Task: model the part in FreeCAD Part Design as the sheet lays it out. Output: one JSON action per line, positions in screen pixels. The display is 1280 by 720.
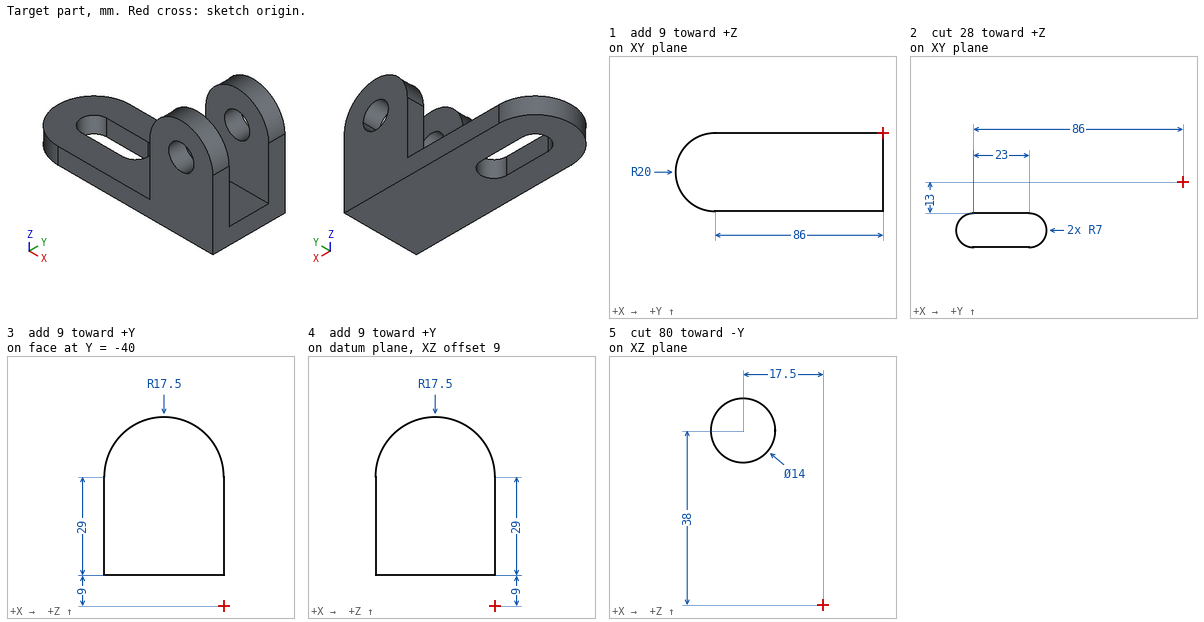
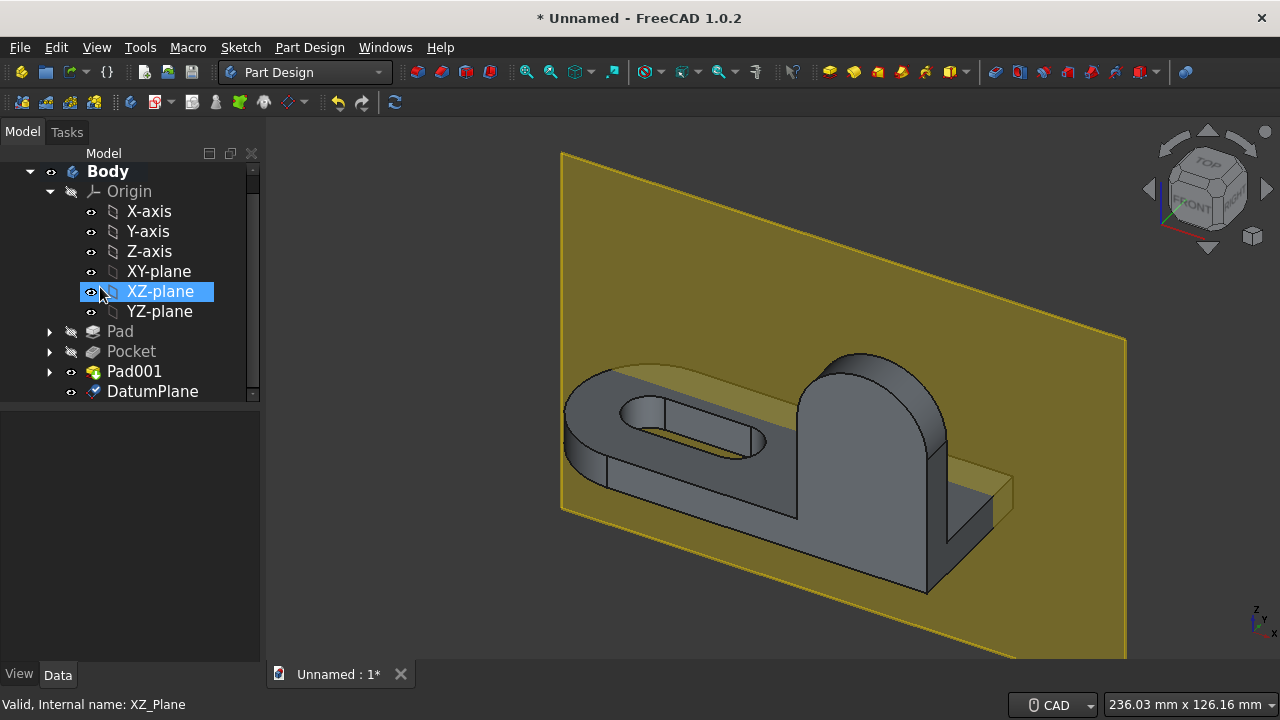
{"action": "left_click", "coordinate": [116, 392]}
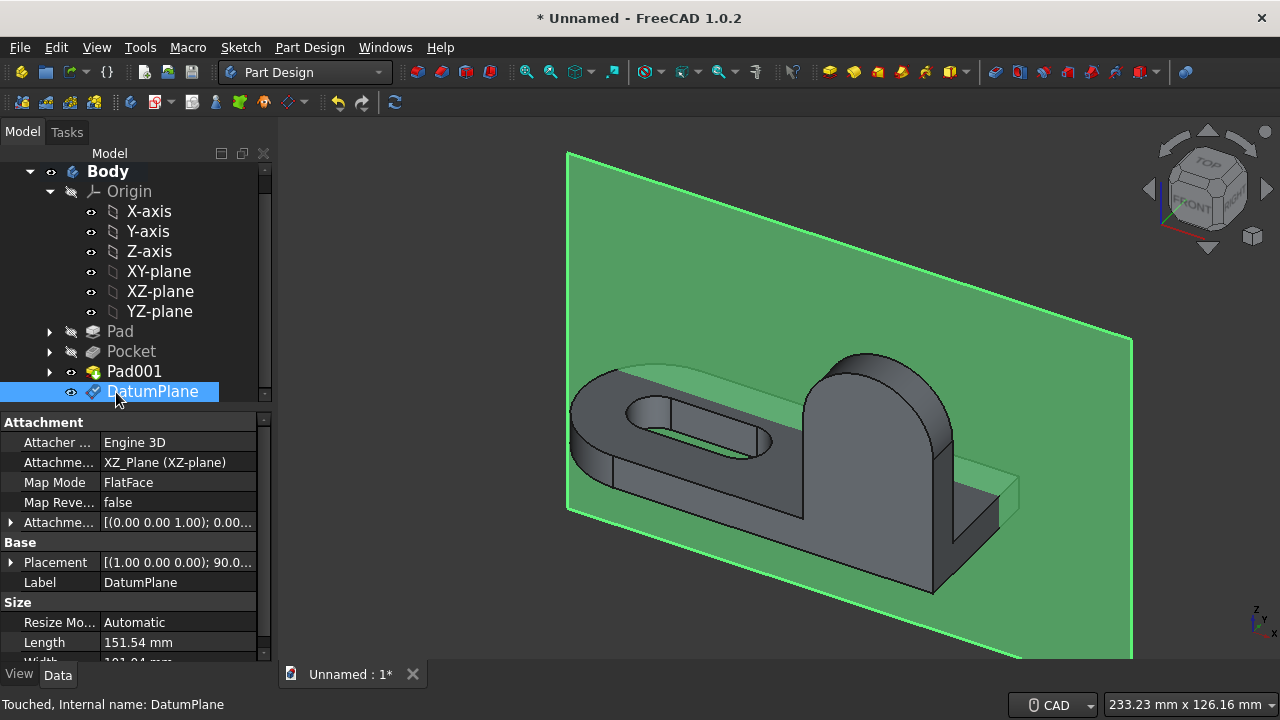
{"action": "left_click", "coordinate": [156, 102]}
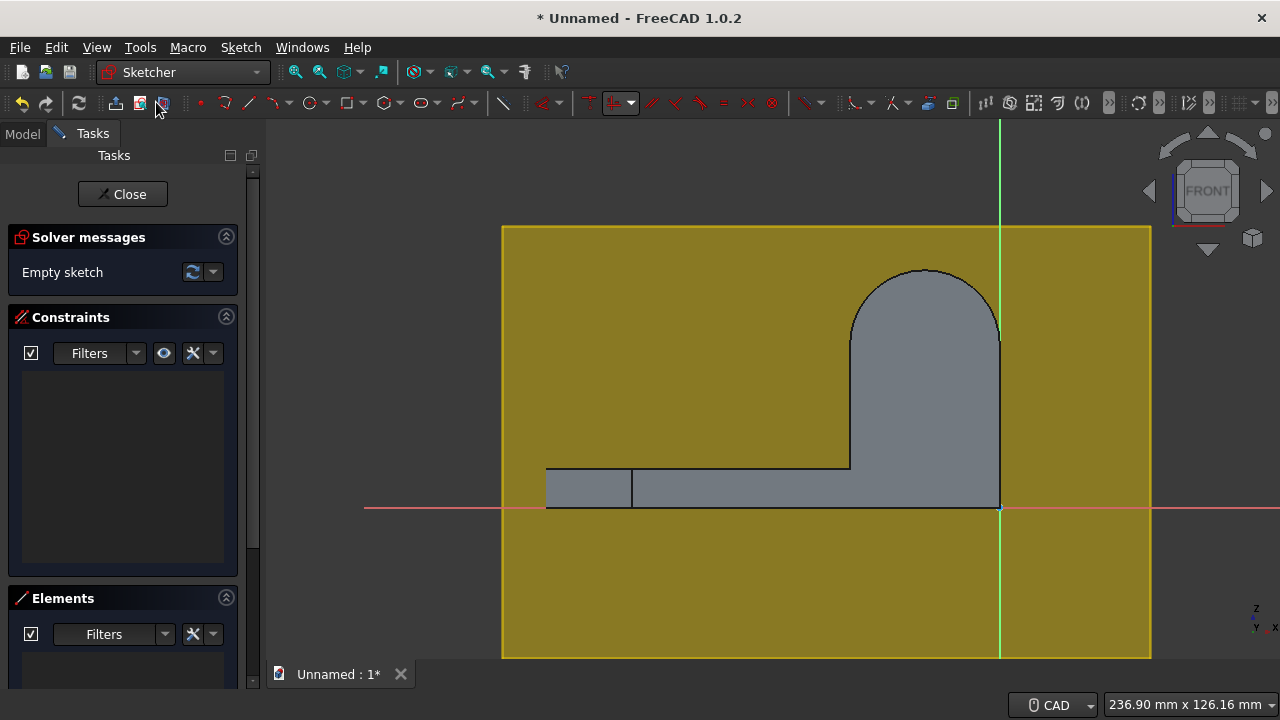
{"action": "left_click", "coordinate": [164, 104]}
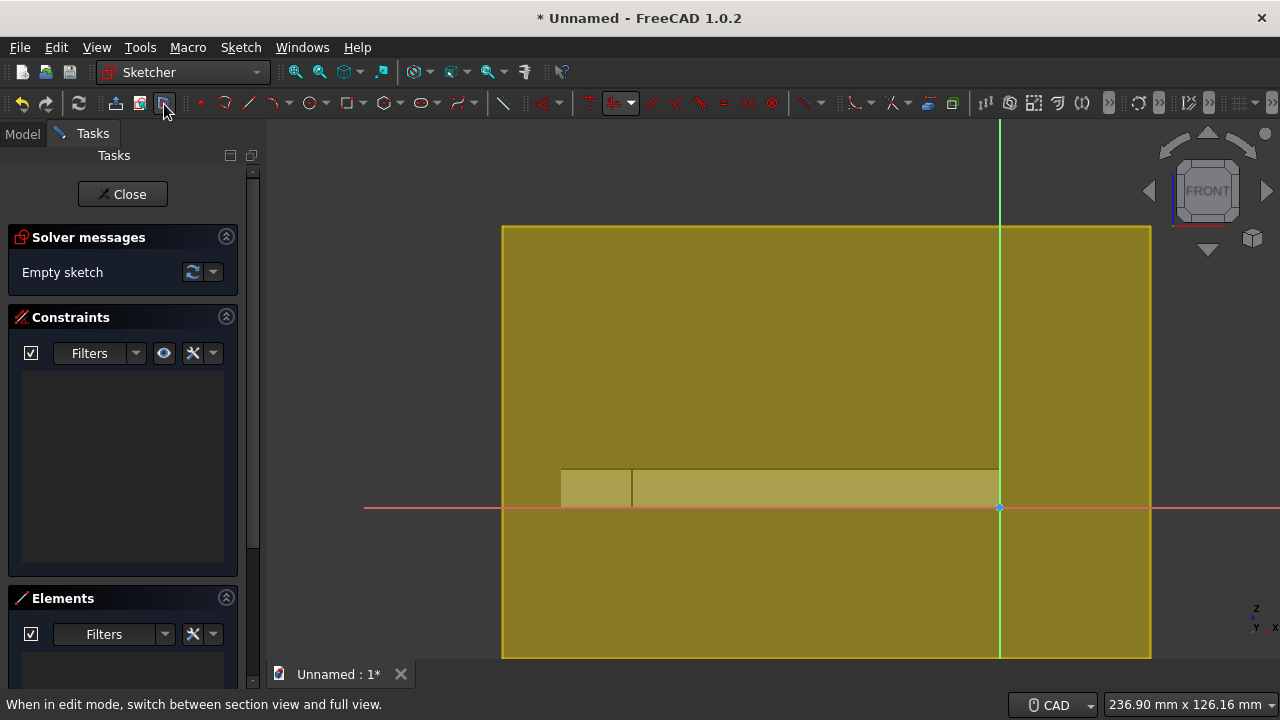
{"action": "scroll", "coordinate": [1115, 389], "scroll_direction": "up", "scroll_amount": 2}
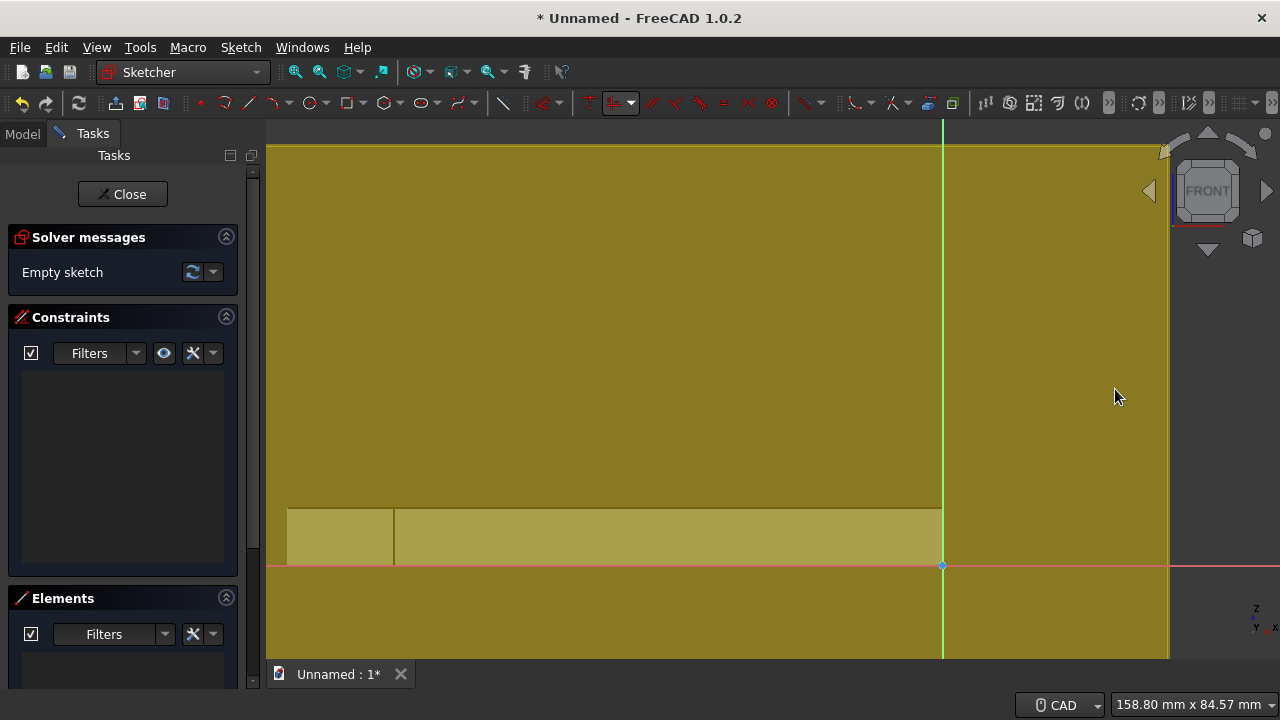
{"action": "left_click", "coordinate": [226, 104]}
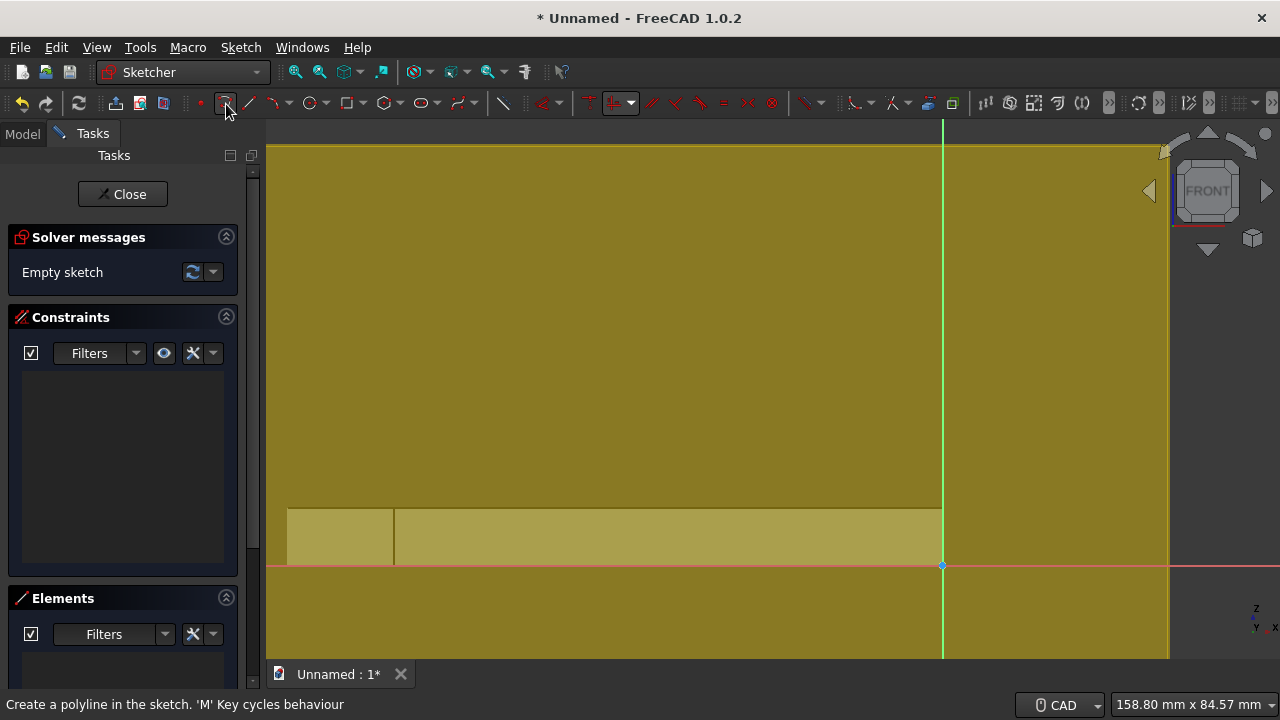
{"action": "left_click", "coordinate": [943, 323]}
{"action": "left_click", "coordinate": [934, 508]}
{"action": "left_click", "coordinate": [719, 508]}
{"action": "left_click", "coordinate": [719, 323]}
{"action": "right_click", "coordinate": [719, 323]}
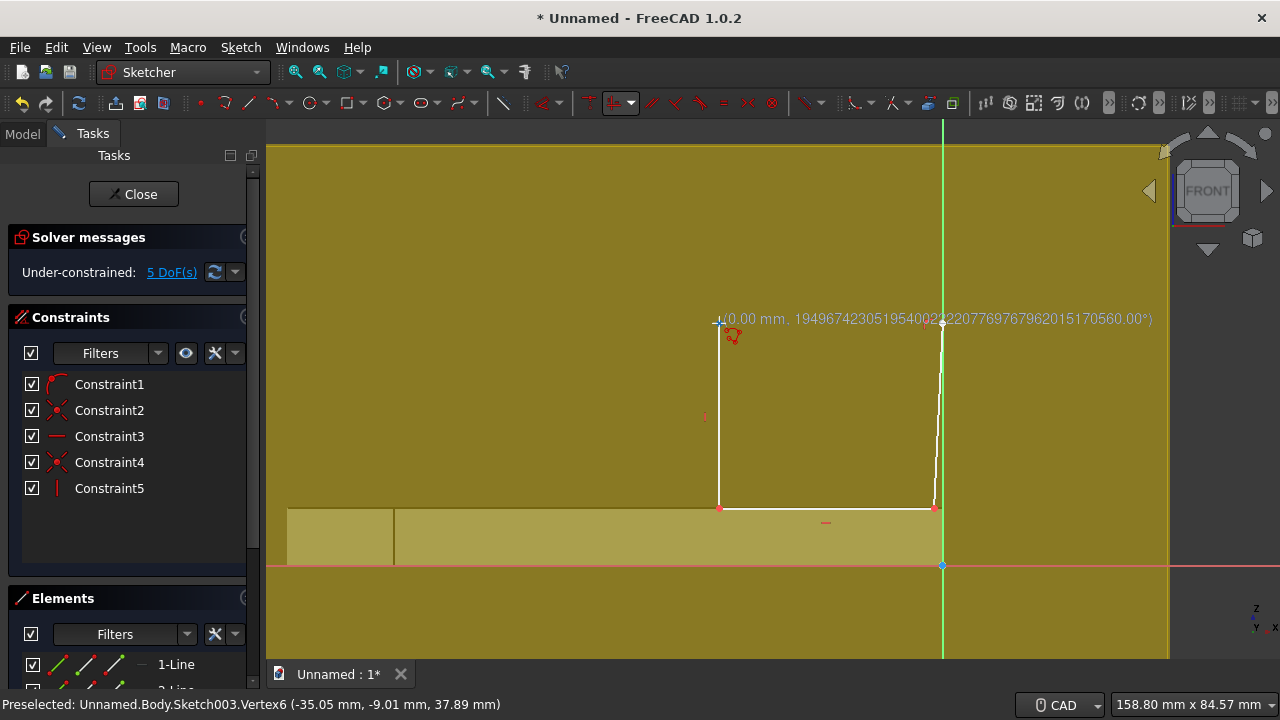
{"action": "left_click", "coordinate": [274, 104]}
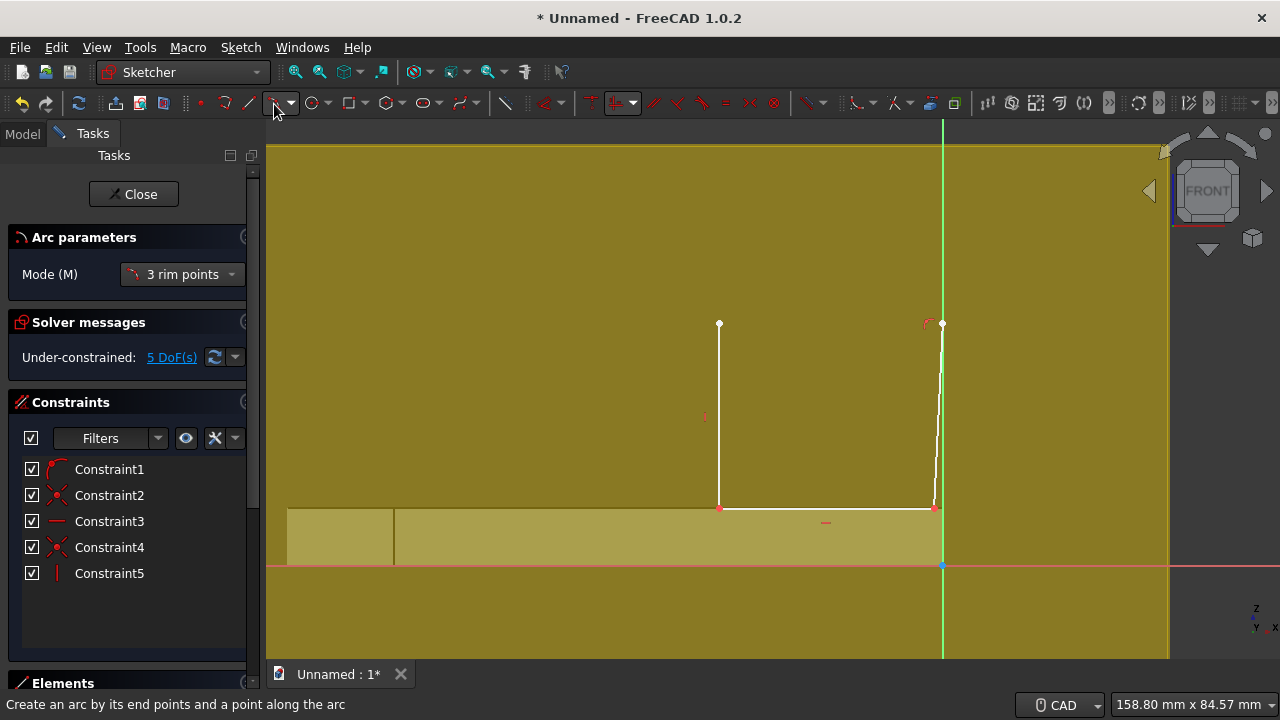
{"action": "left_click", "coordinate": [719, 324]}
{"action": "left_click", "coordinate": [943, 324]}
{"action": "left_click", "coordinate": [831, 212]}
{"action": "key", "text": "Escape"}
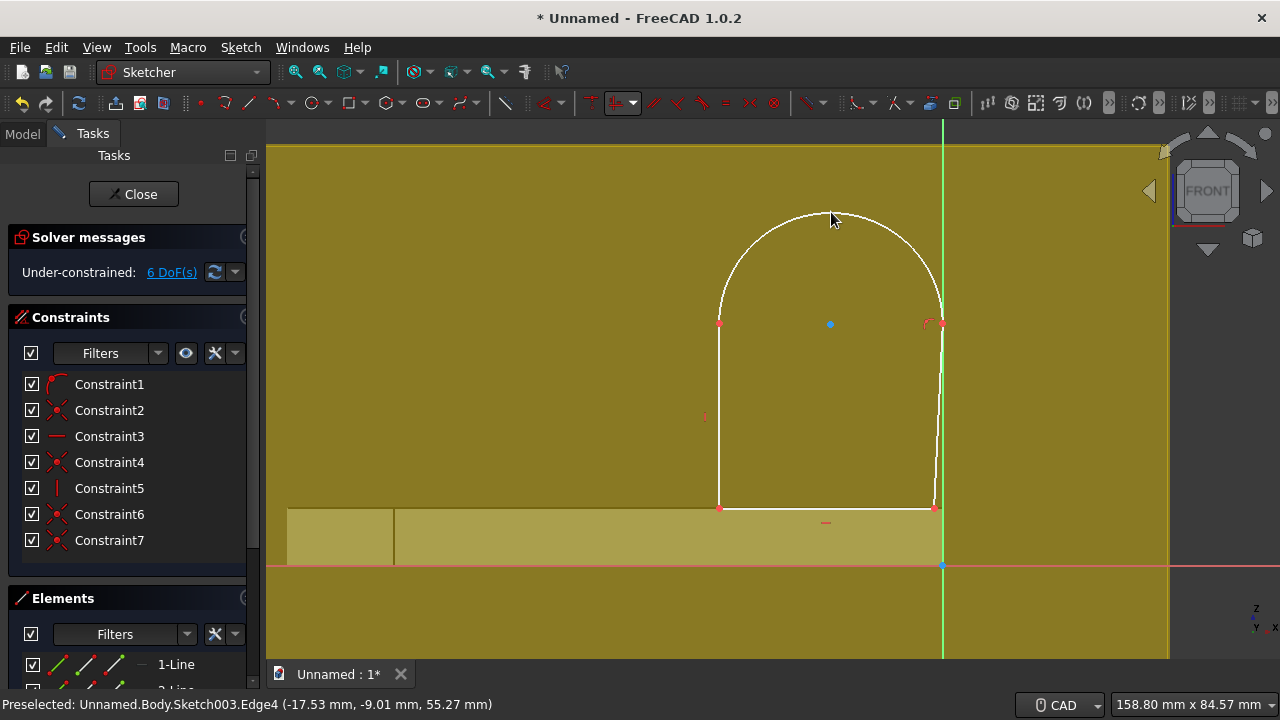
{"action": "left_click", "coordinate": [940, 379]}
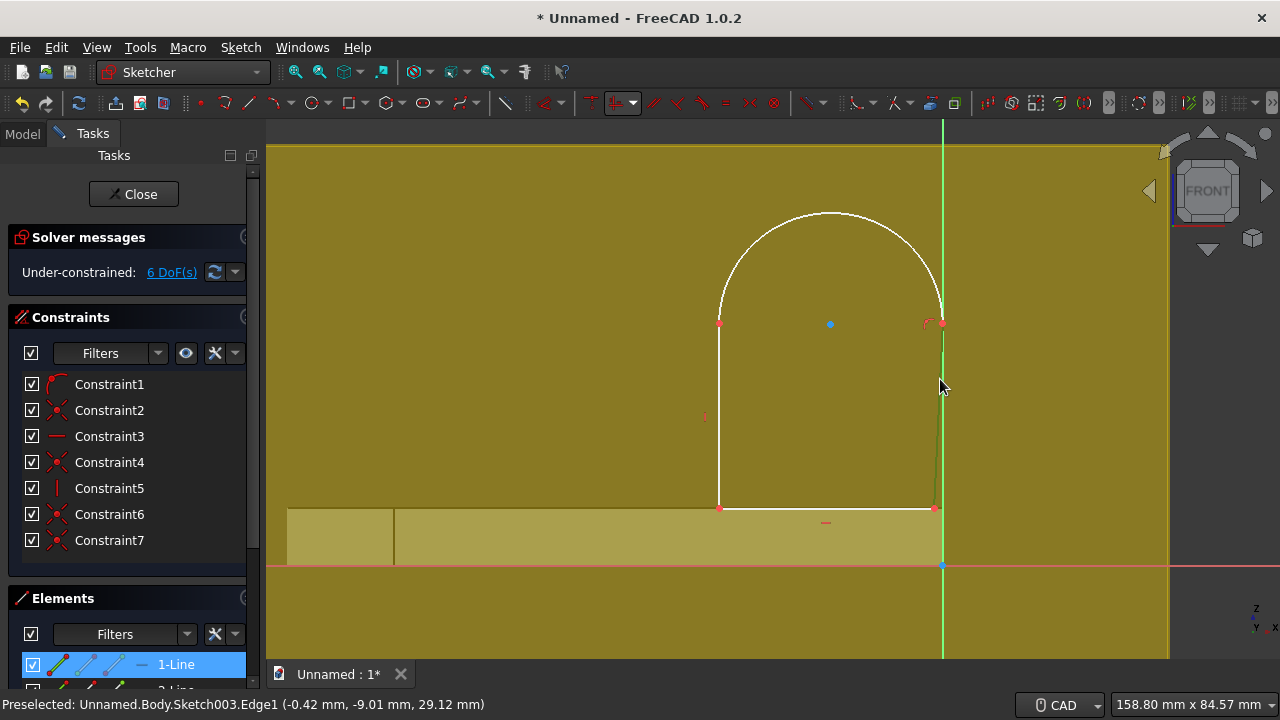
{"action": "left_click", "coordinate": [896, 234]}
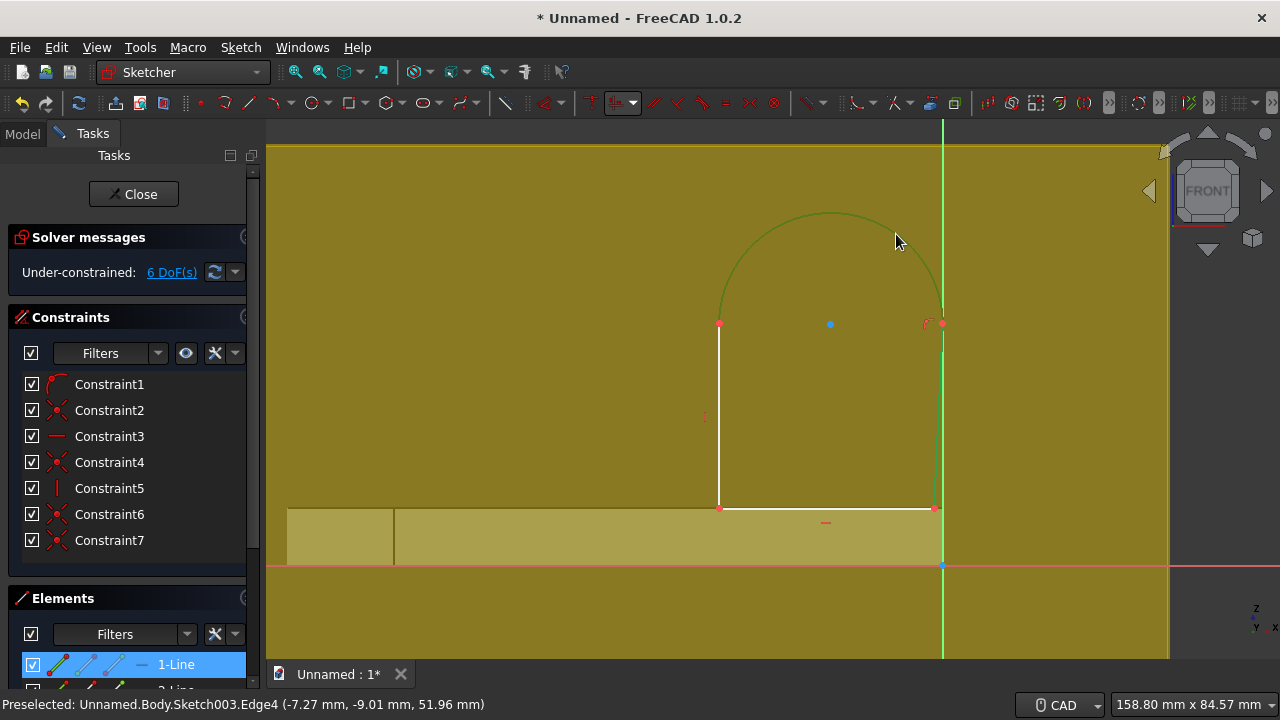
{"action": "left_click", "coordinate": [702, 104]}